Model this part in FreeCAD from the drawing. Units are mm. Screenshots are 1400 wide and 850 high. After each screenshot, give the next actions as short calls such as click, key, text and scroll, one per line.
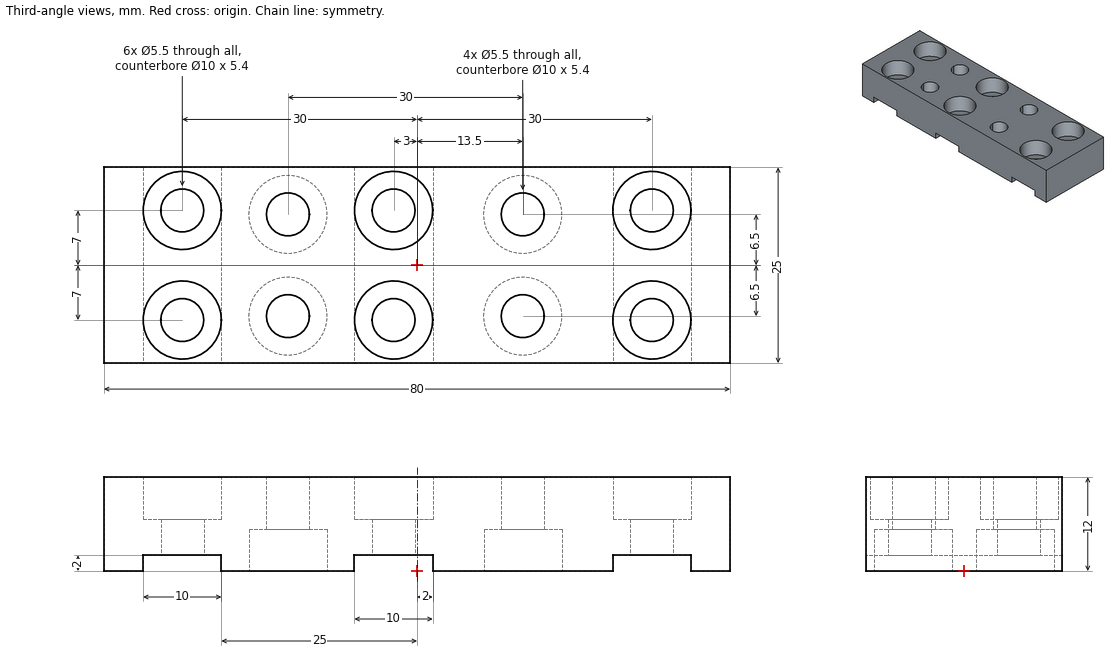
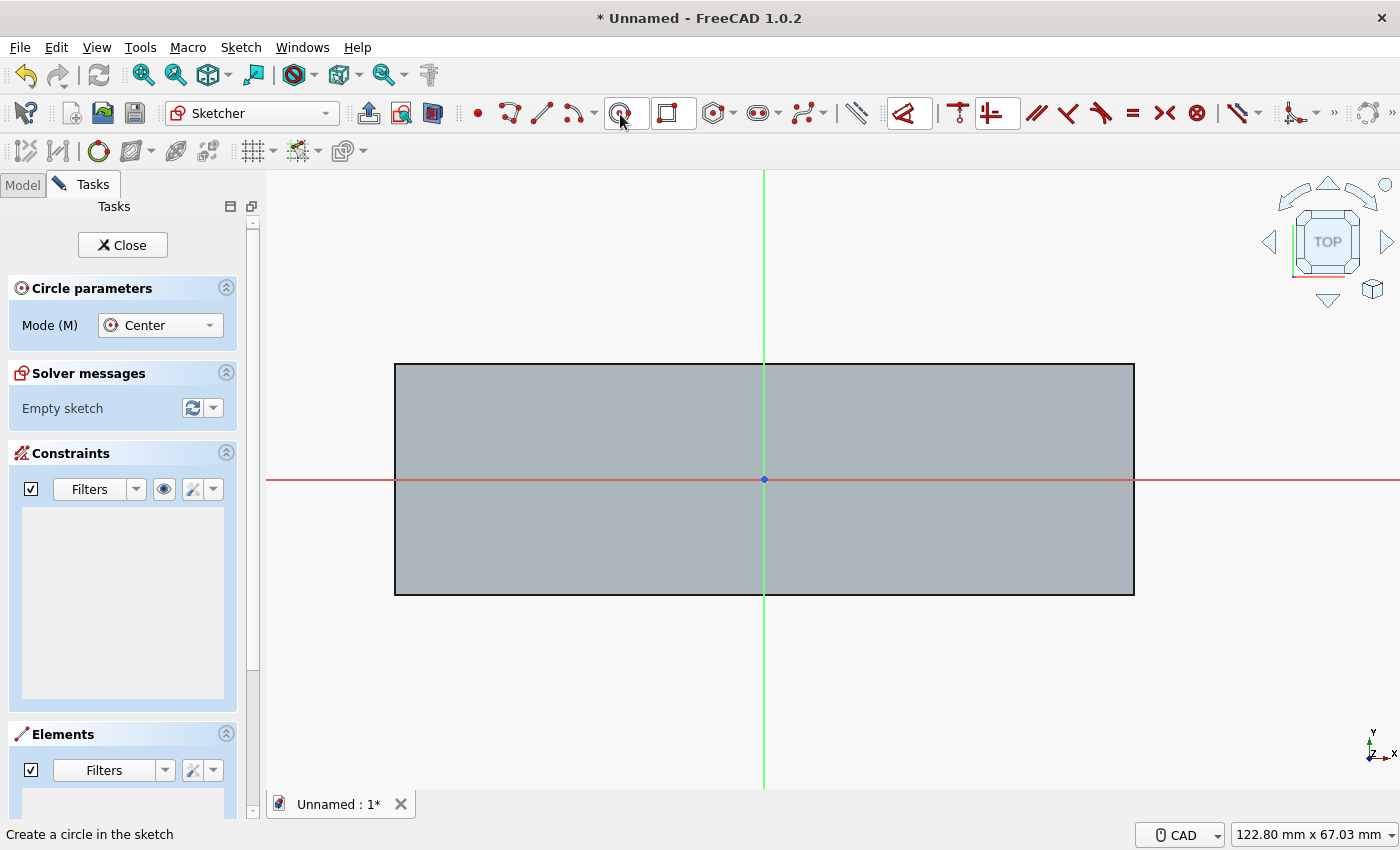
click(487, 415)
click(505, 397)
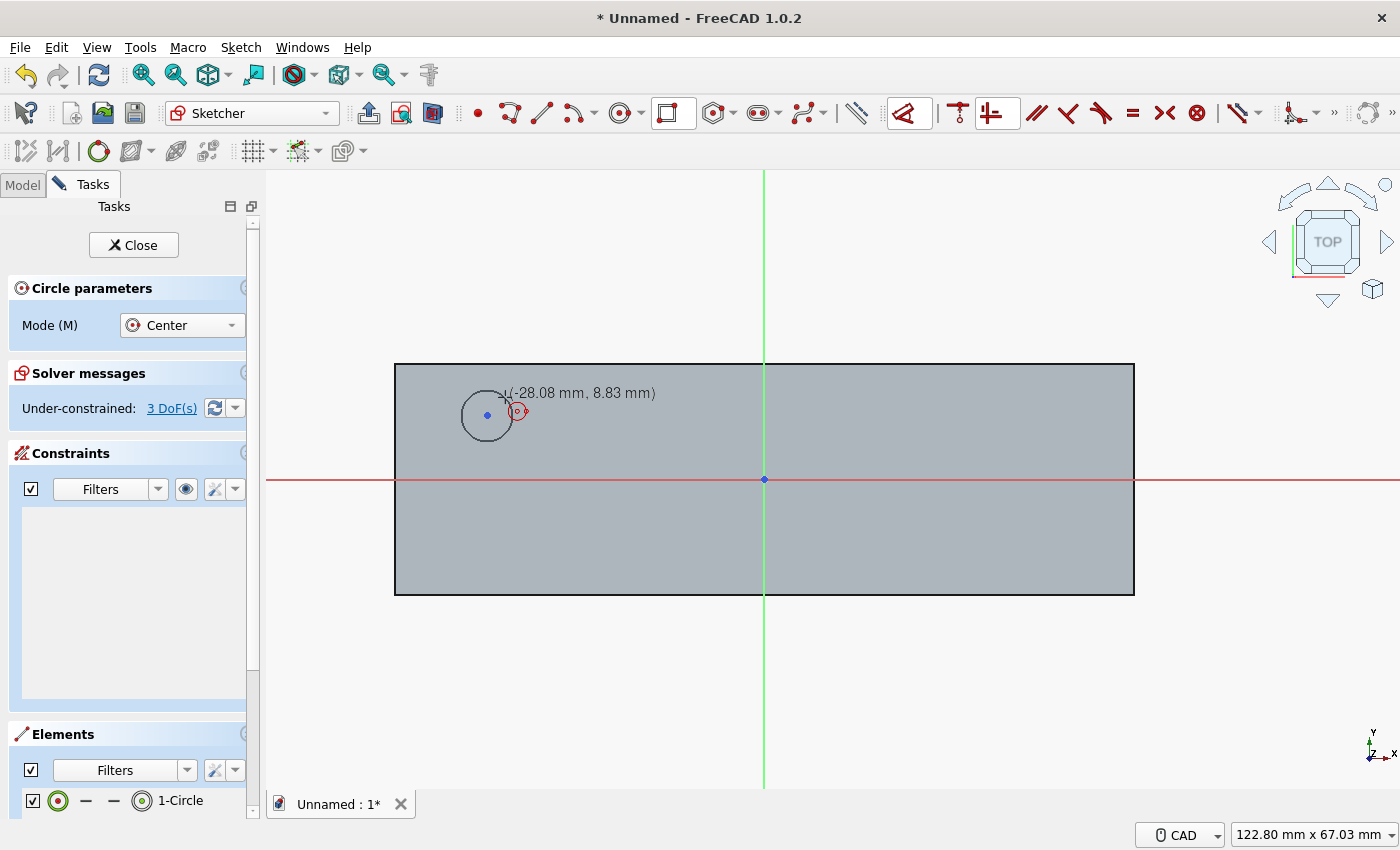
click(487, 544)
click(505, 526)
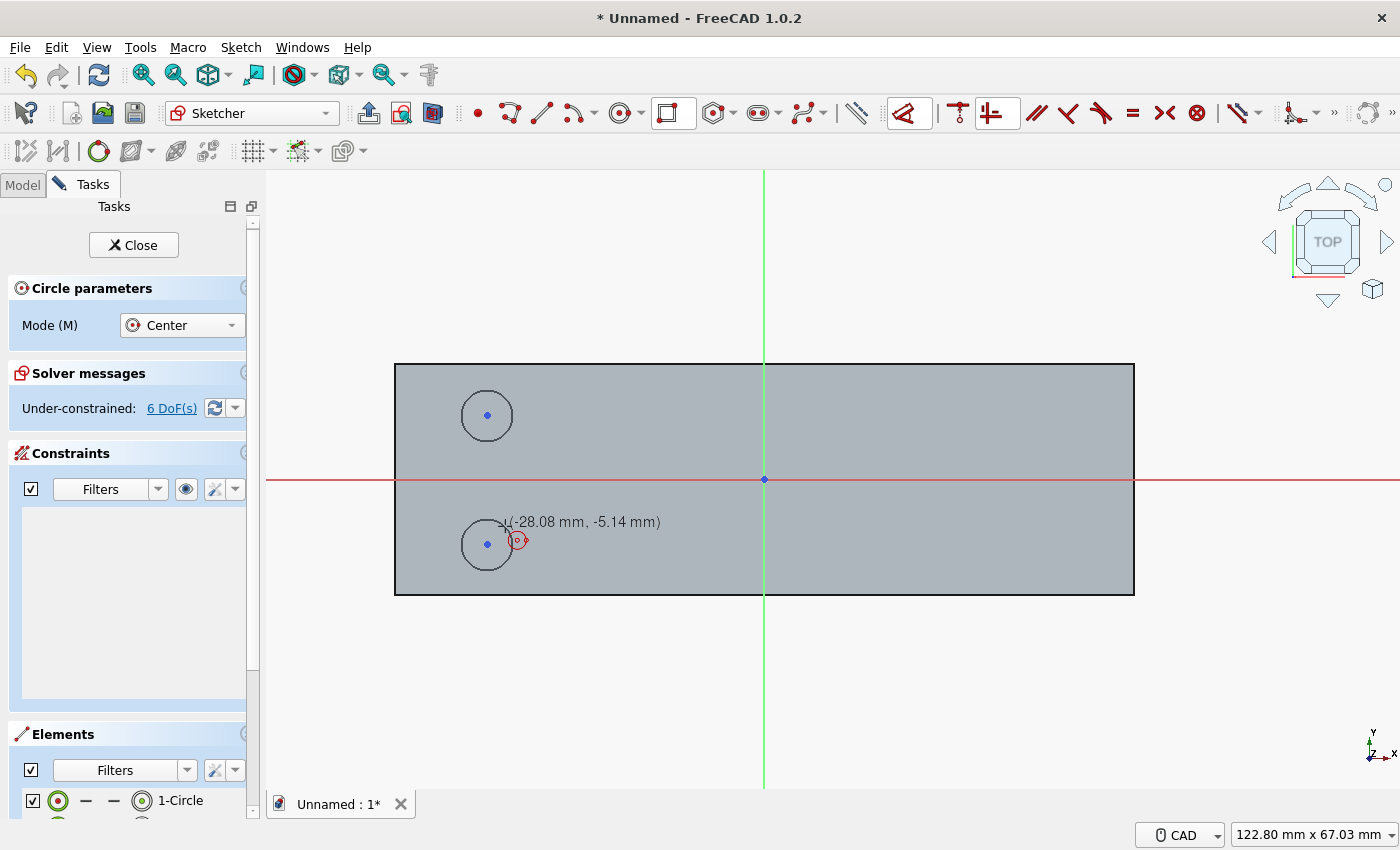
click(737, 415)
click(719, 397)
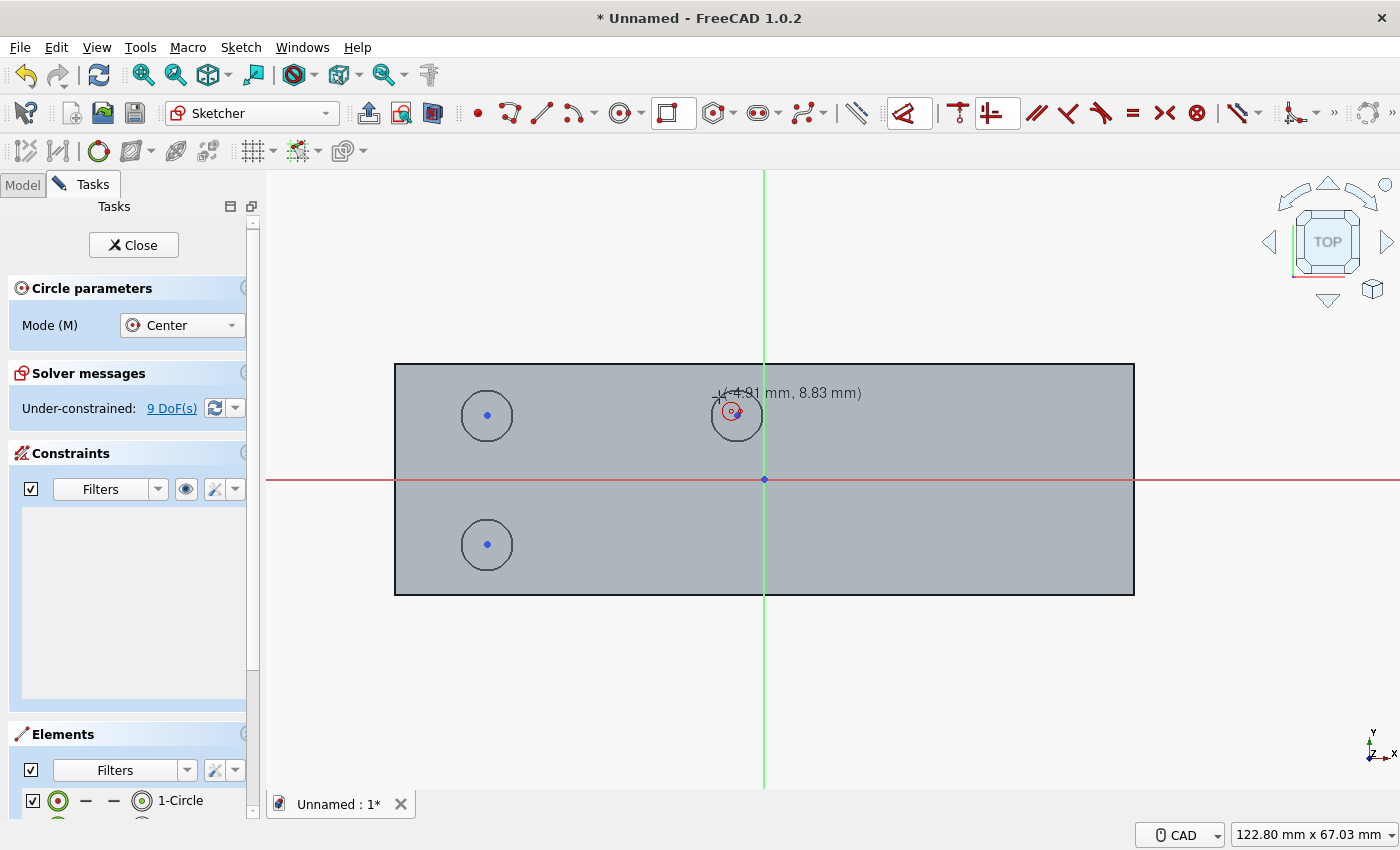
click(737, 544)
click(719, 526)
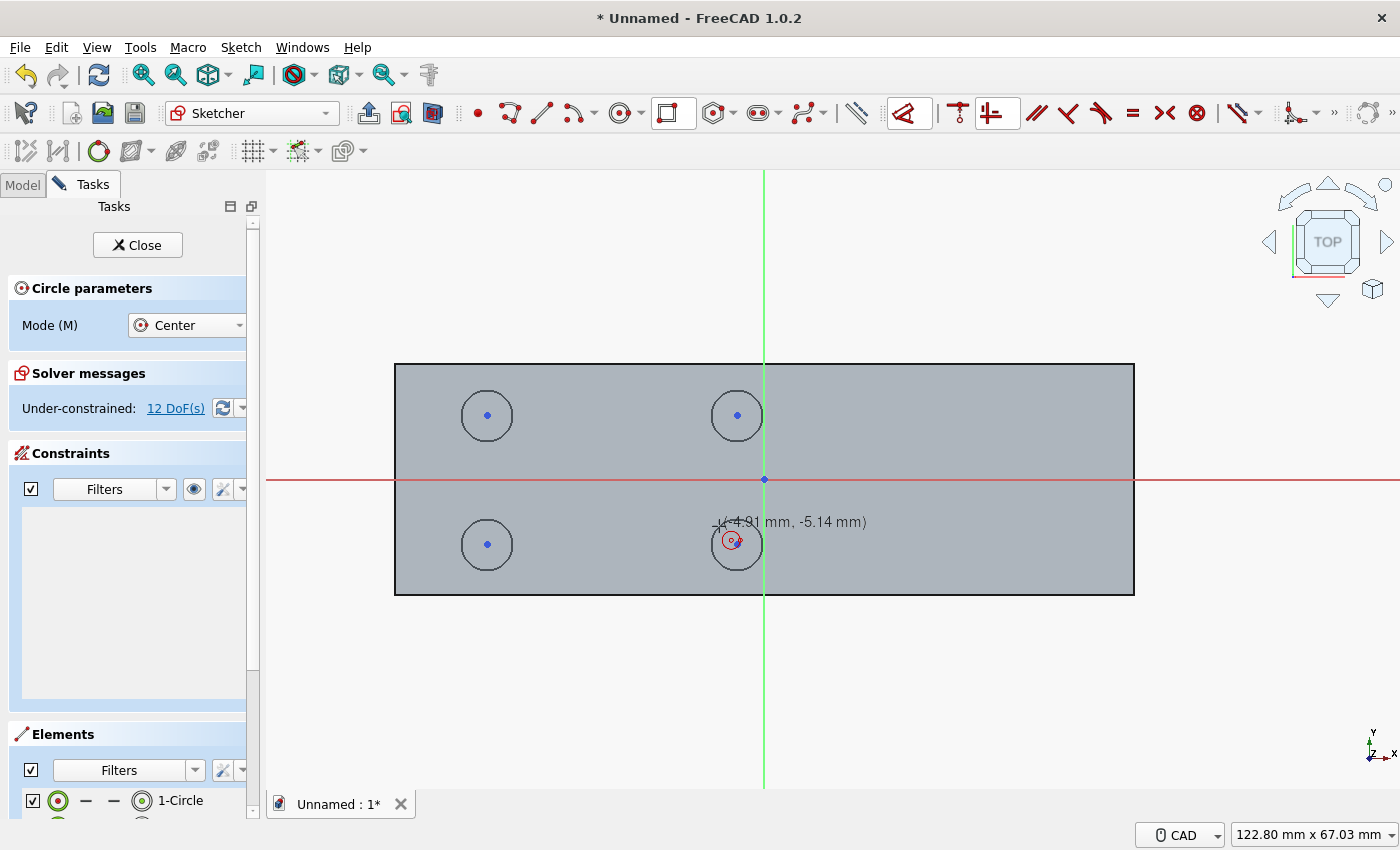
click(1041, 415)
click(1059, 397)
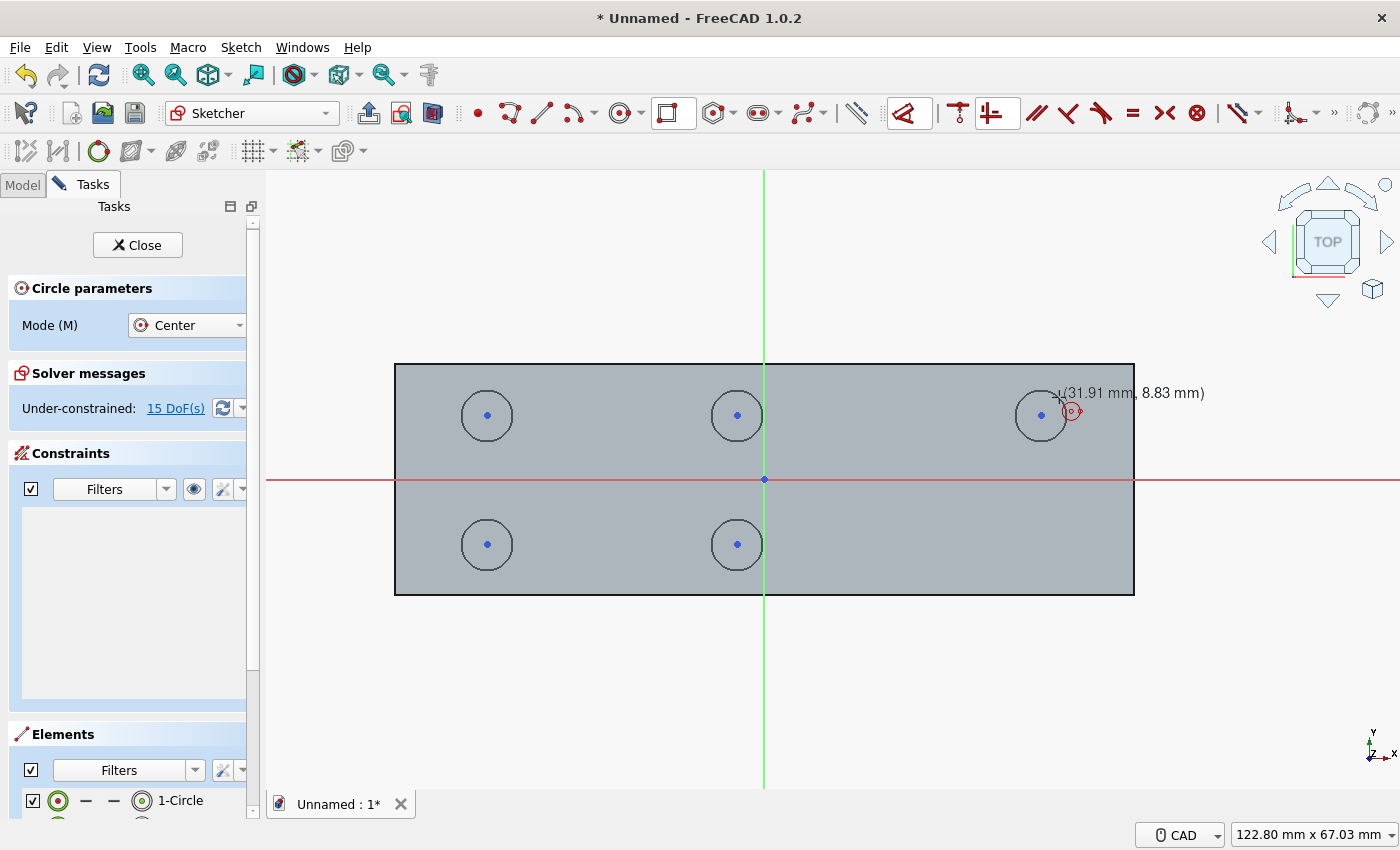
click(1041, 544)
click(1059, 526)
key(Escape)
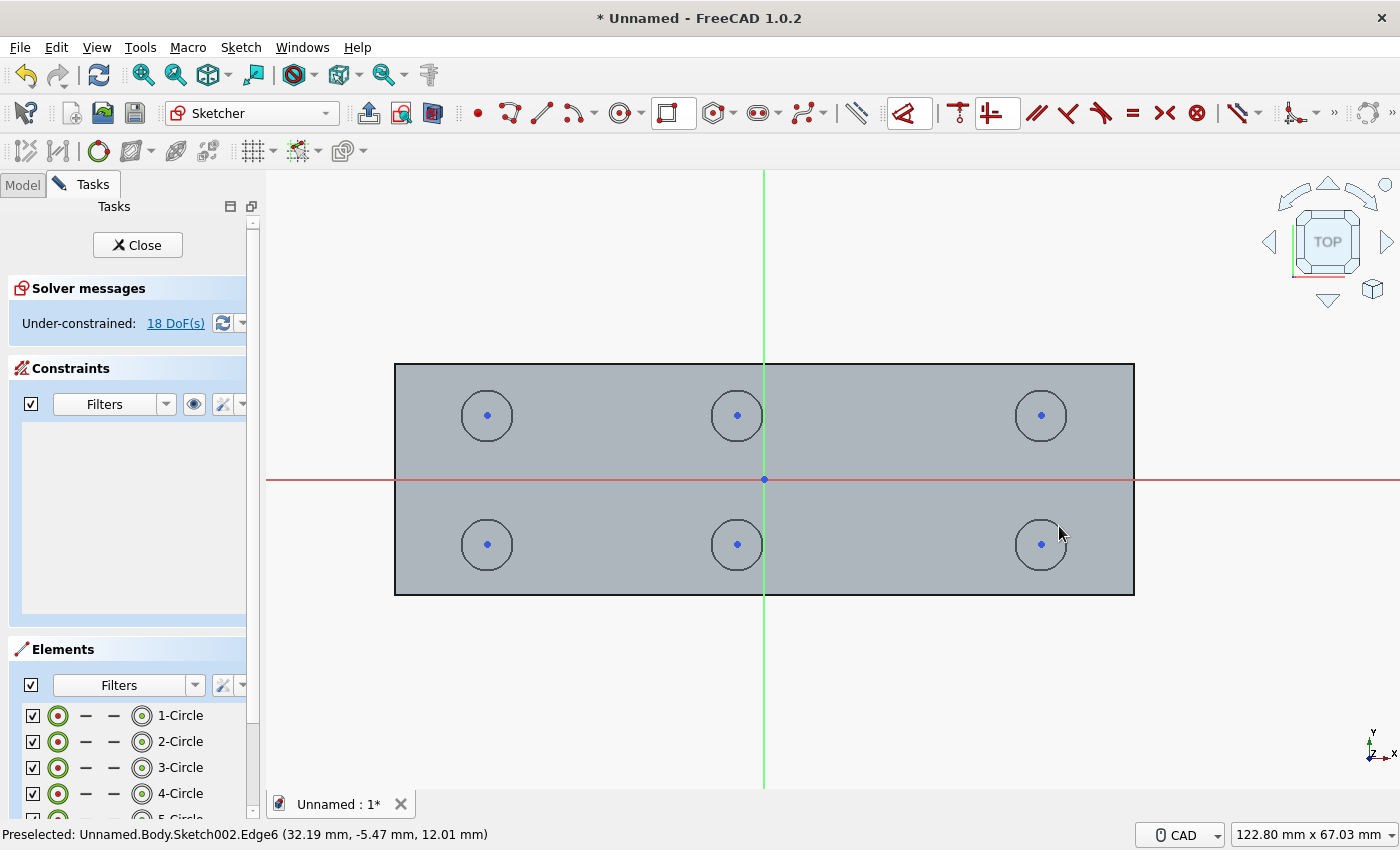
click(505, 398)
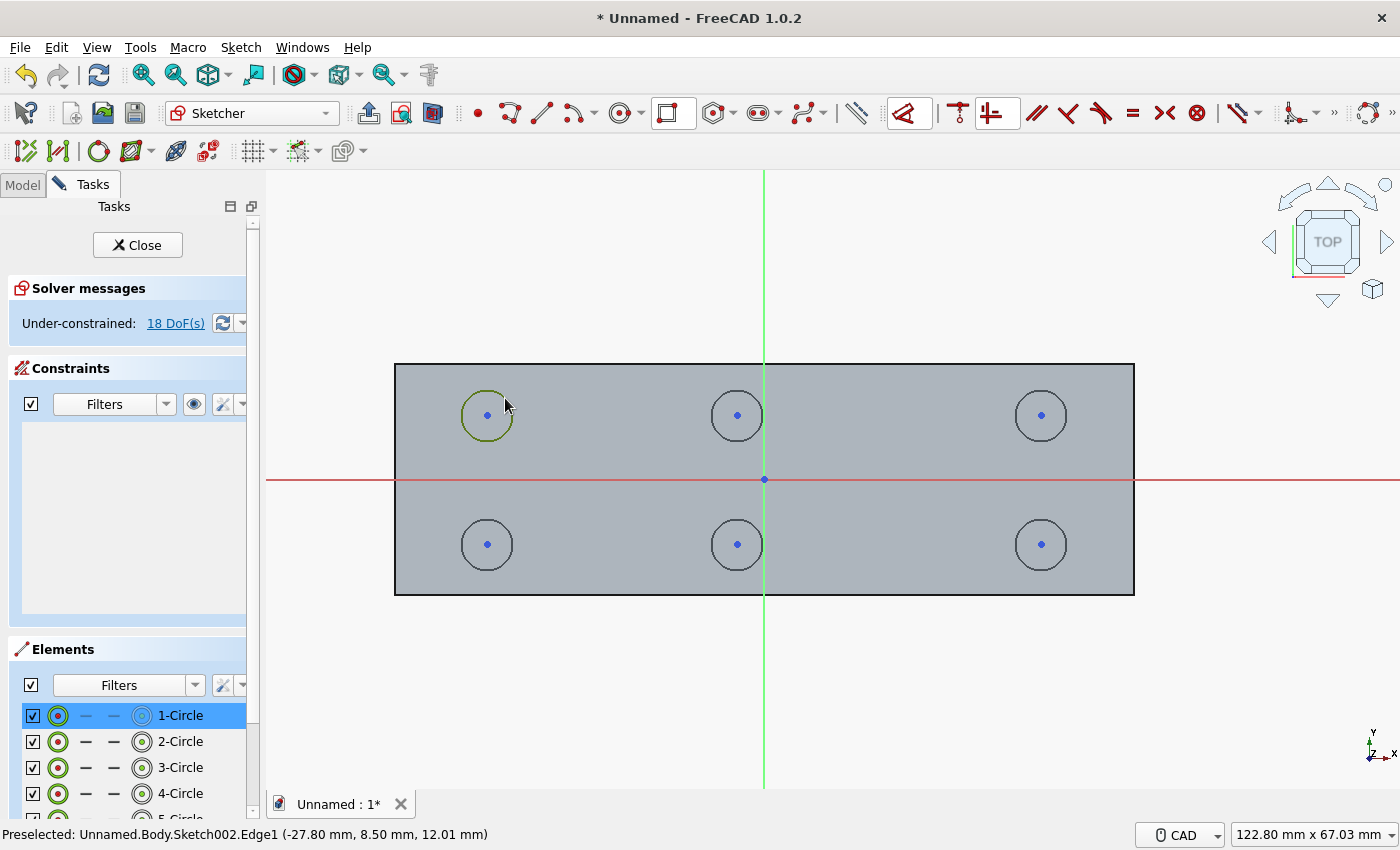
click(505, 527)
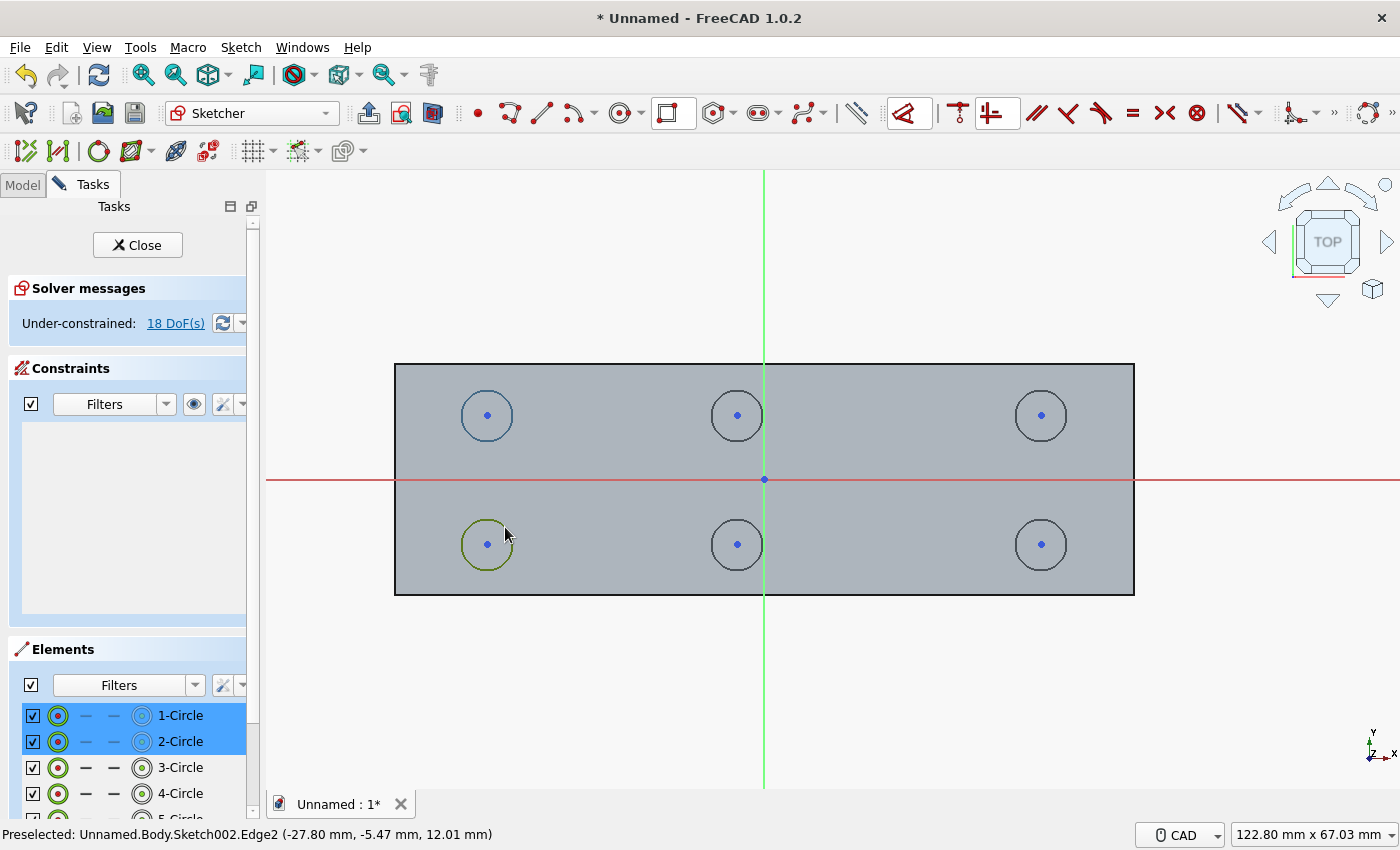
scroll(755, 398, up, 2)